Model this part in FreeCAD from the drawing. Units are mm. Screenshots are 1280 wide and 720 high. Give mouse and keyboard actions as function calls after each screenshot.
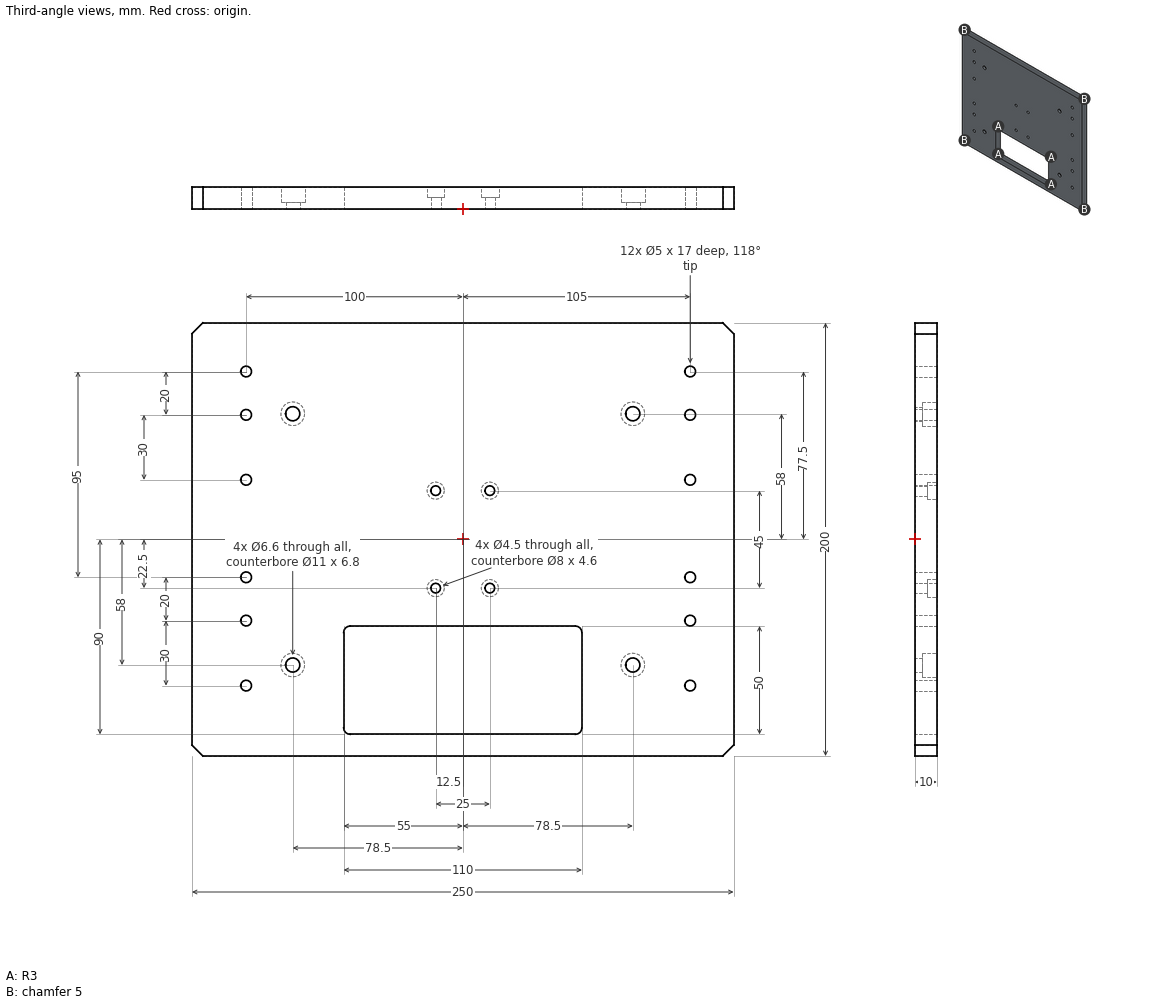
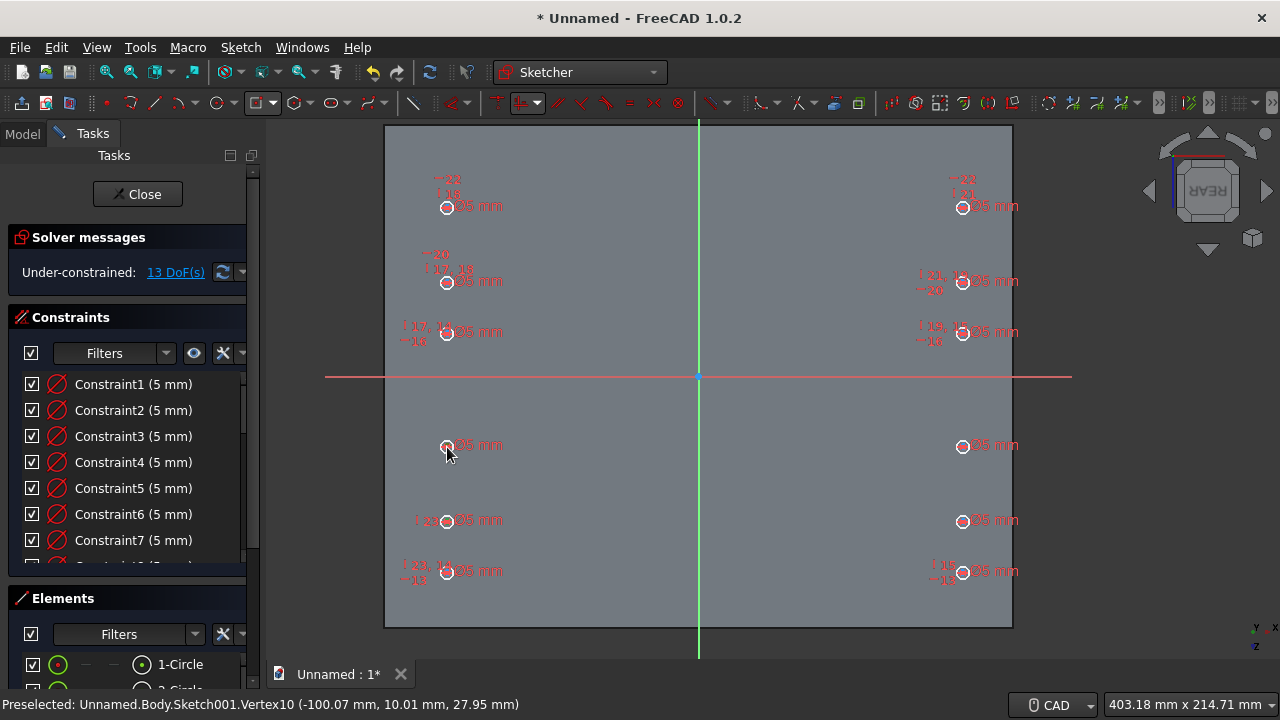
click(540, 104)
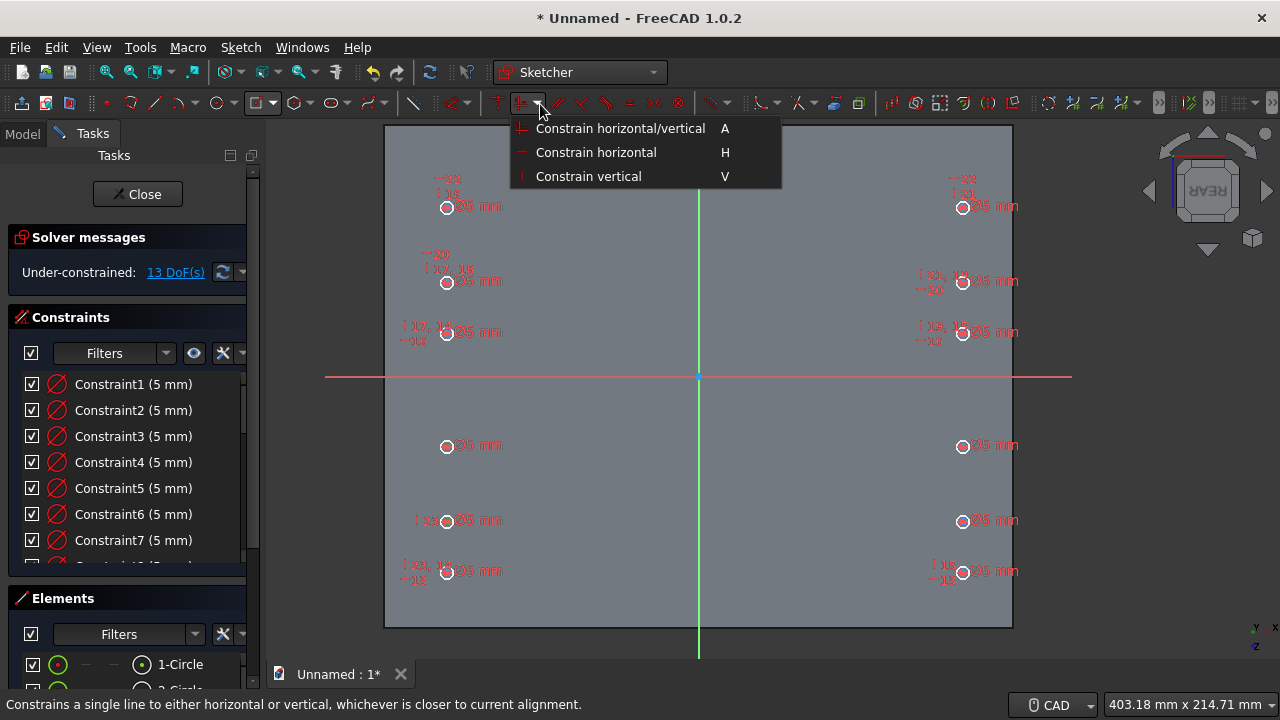
click(646, 176)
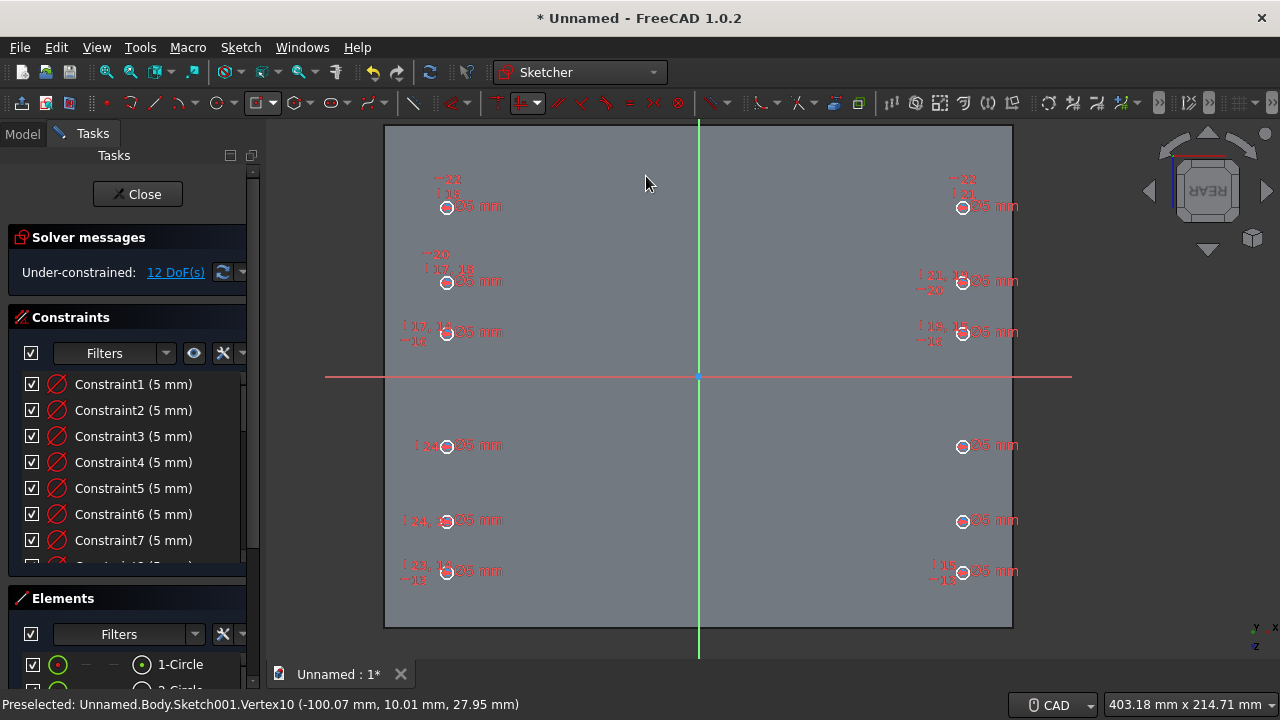
click(963, 573)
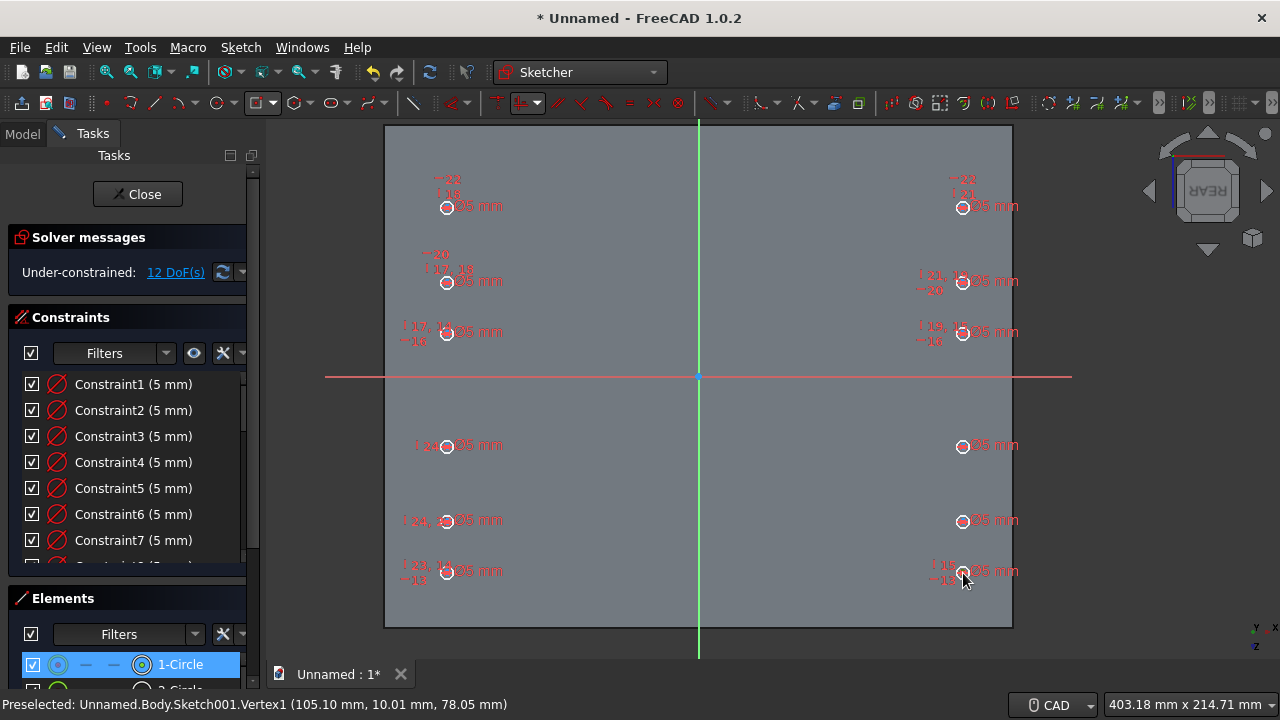
click(963, 522)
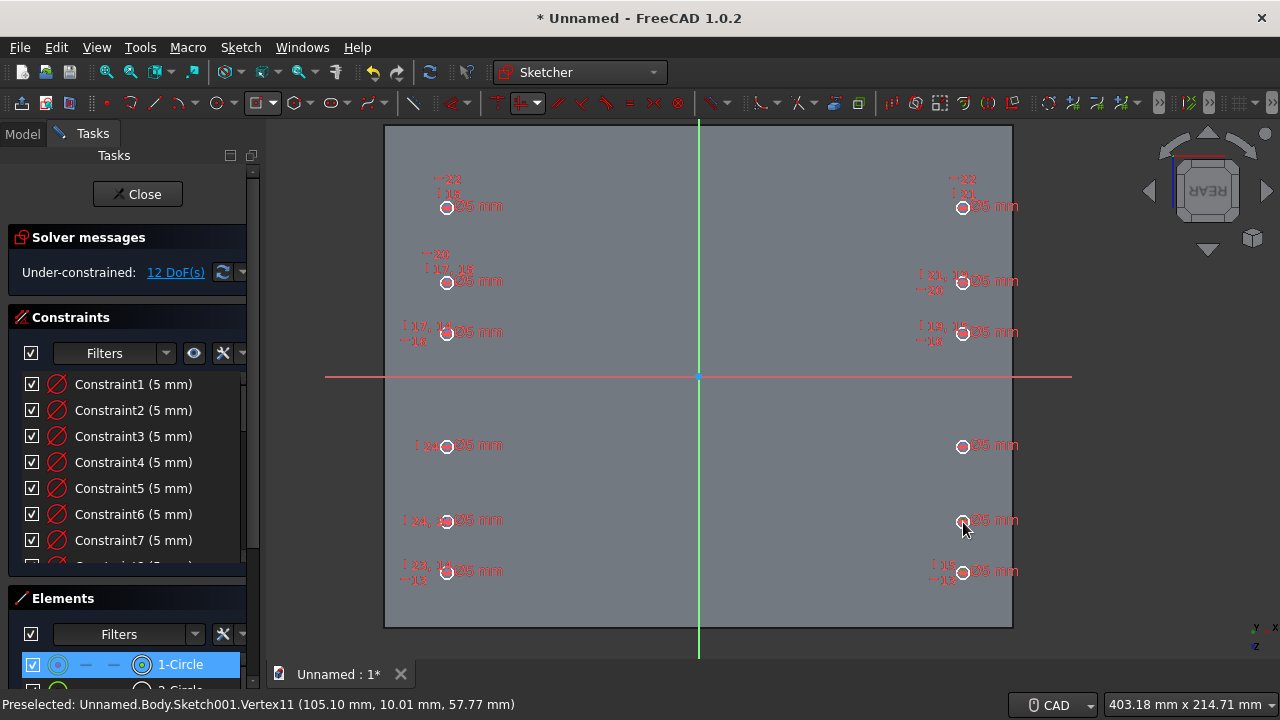
click(540, 104)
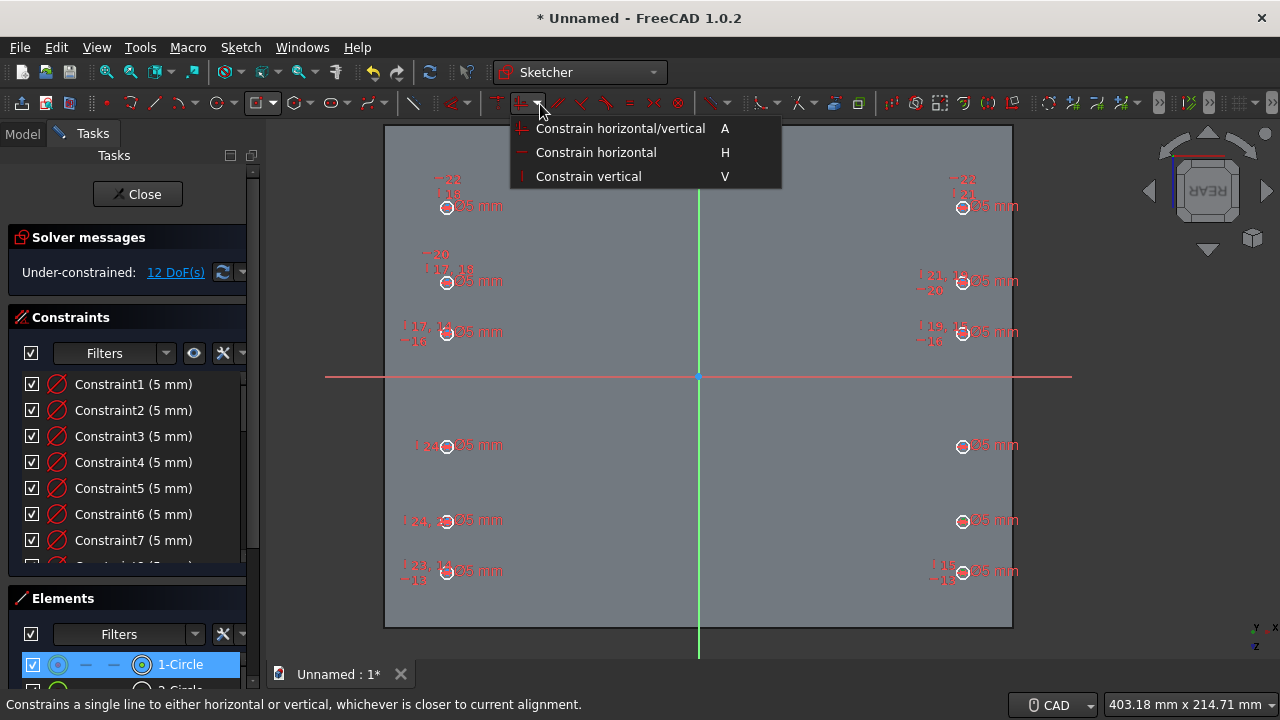
click(646, 176)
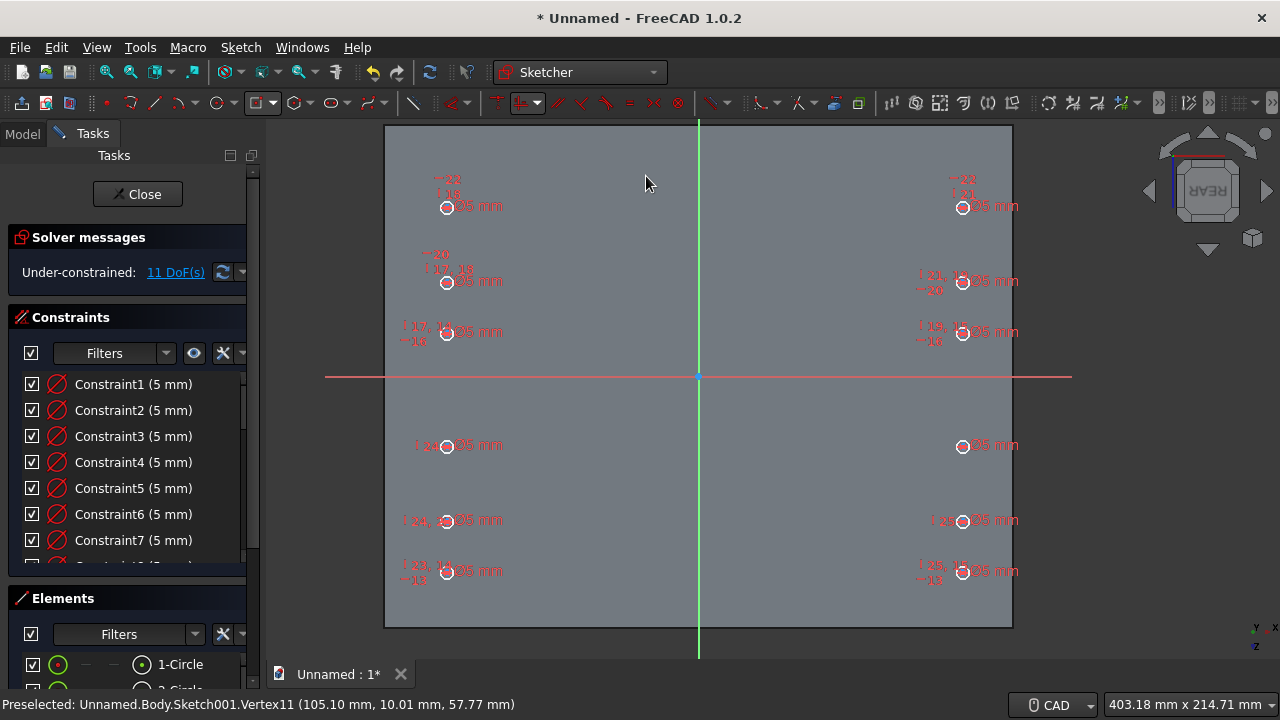
click(447, 522)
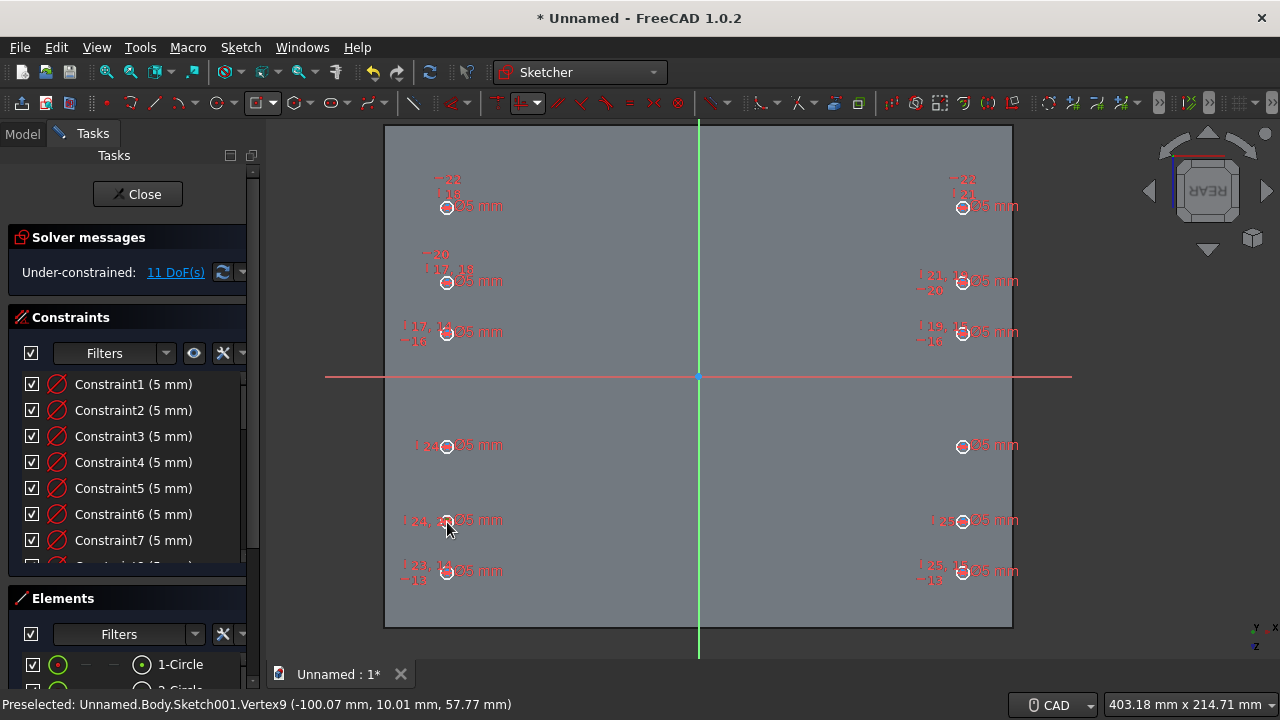
click(963, 522)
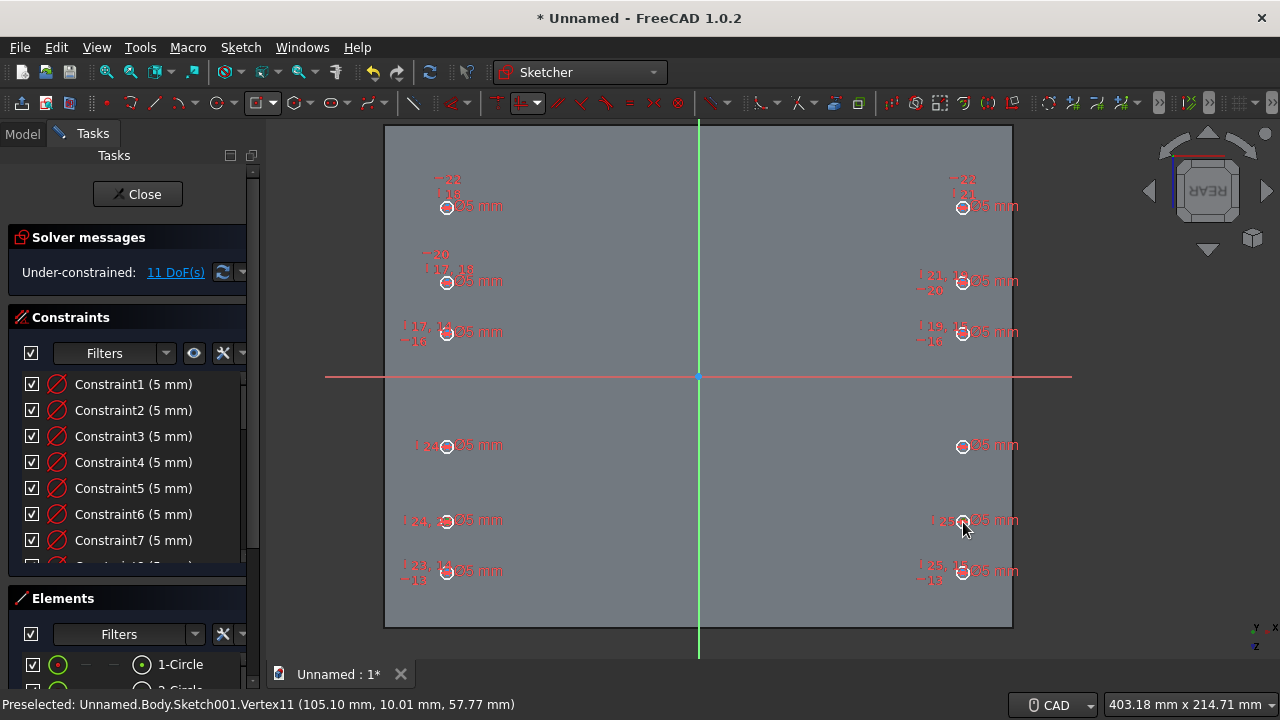
click(540, 104)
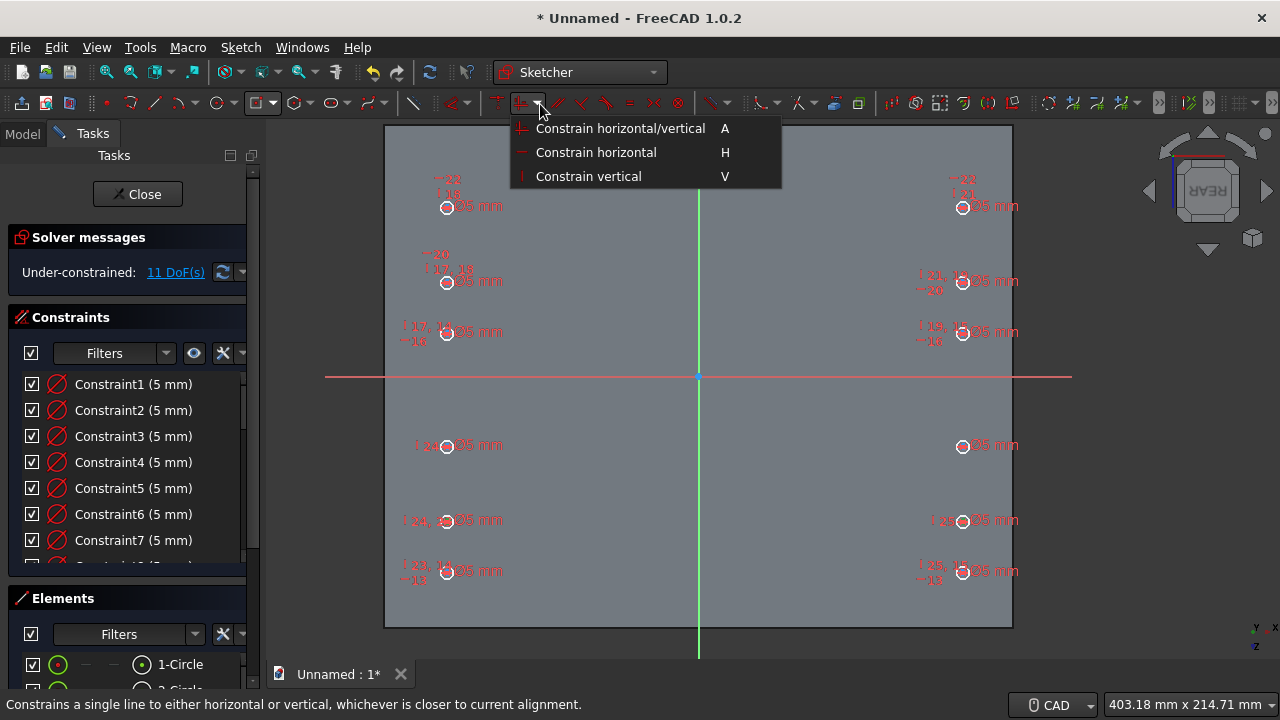
click(646, 152)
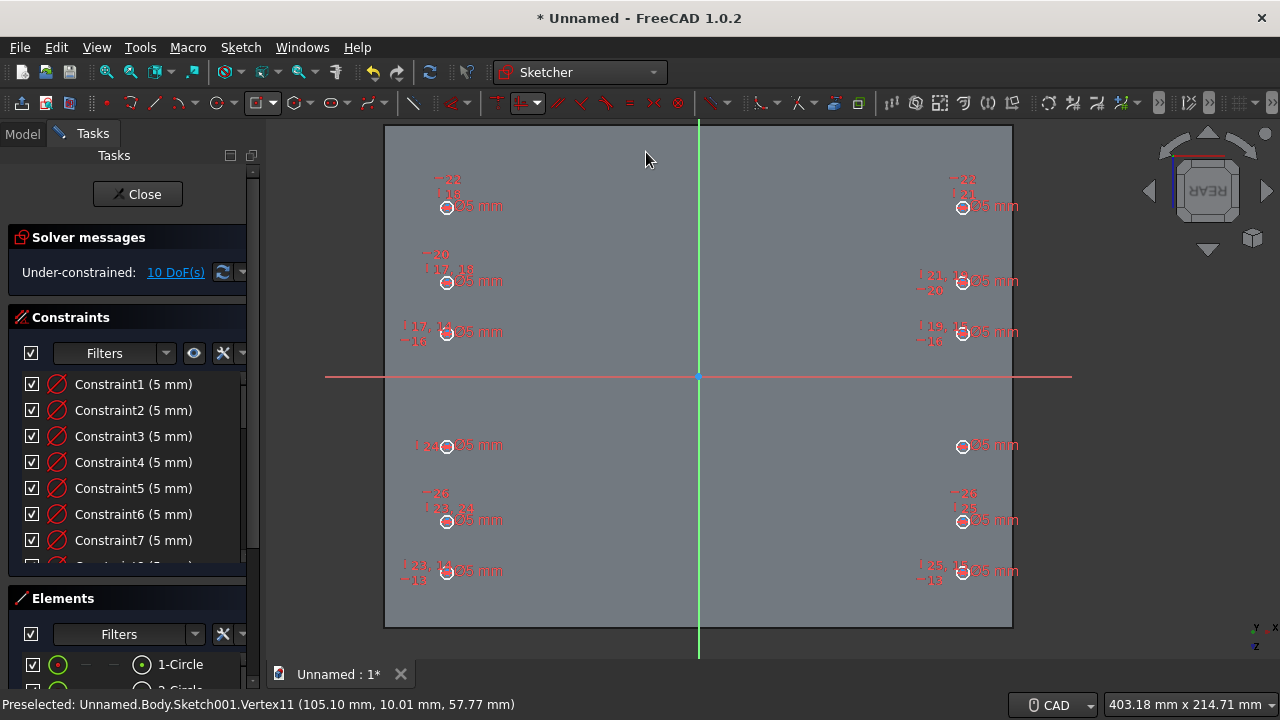
click(963, 522)